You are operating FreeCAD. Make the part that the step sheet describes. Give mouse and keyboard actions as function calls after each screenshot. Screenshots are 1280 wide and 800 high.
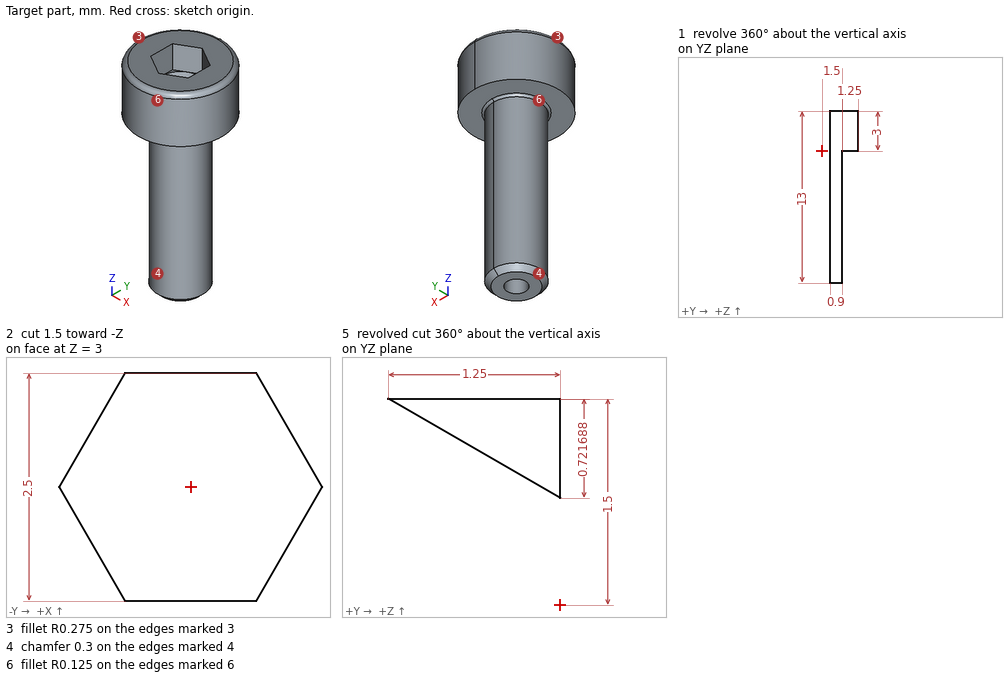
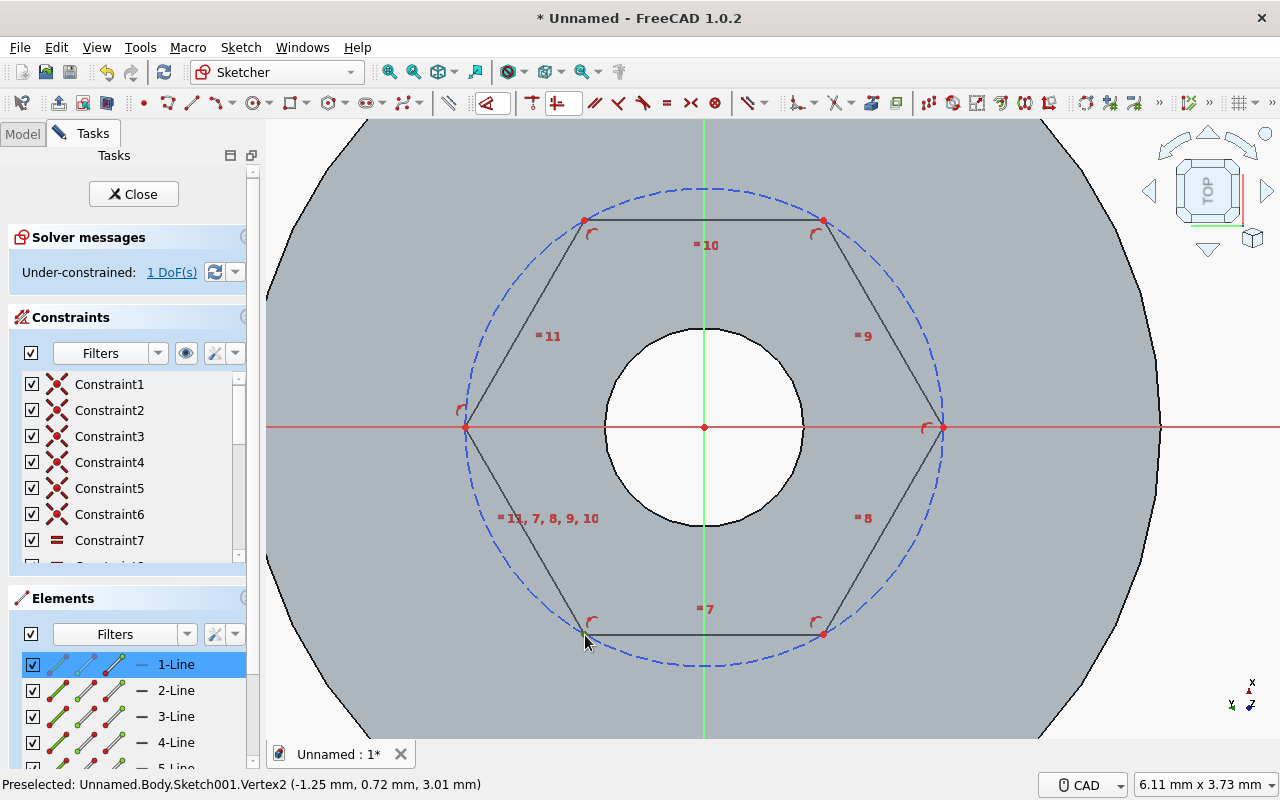
click(824, 220)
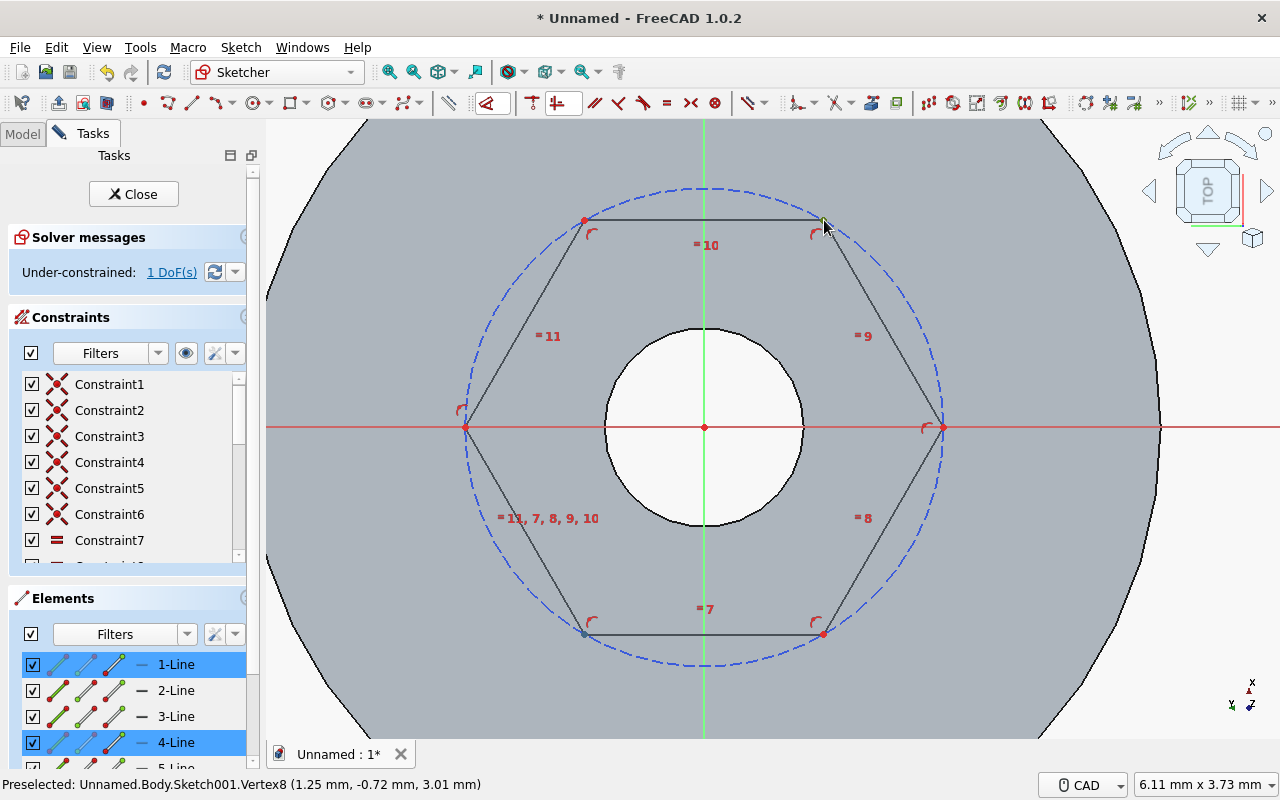
click(504, 104)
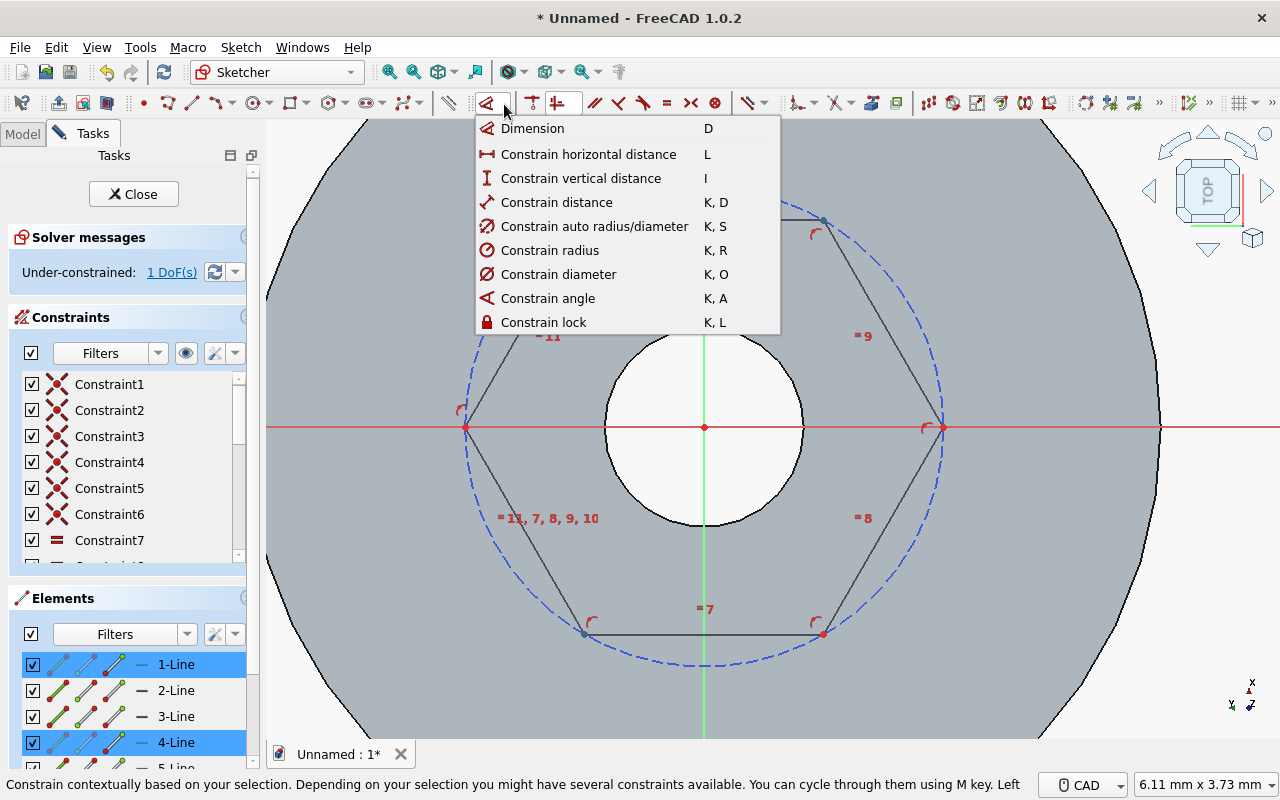
click(628, 178)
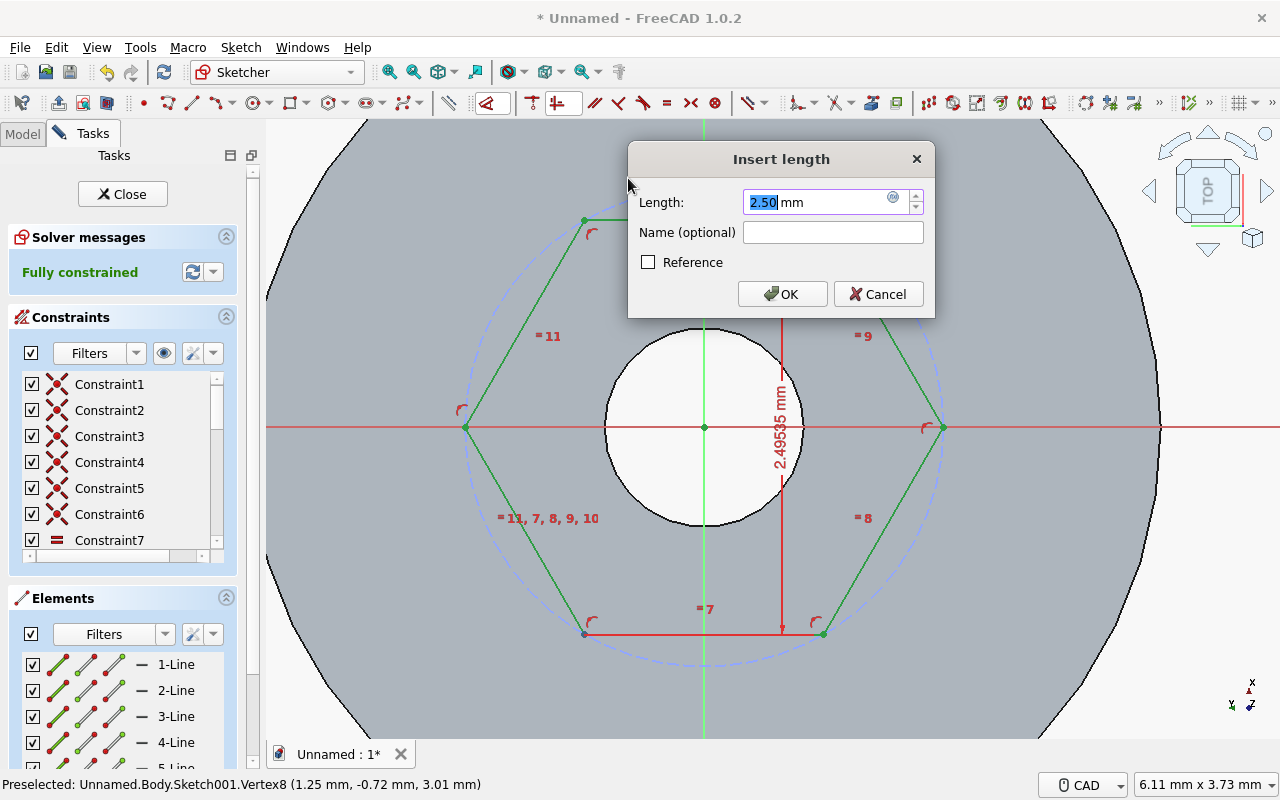
text(2.5)
key(Return)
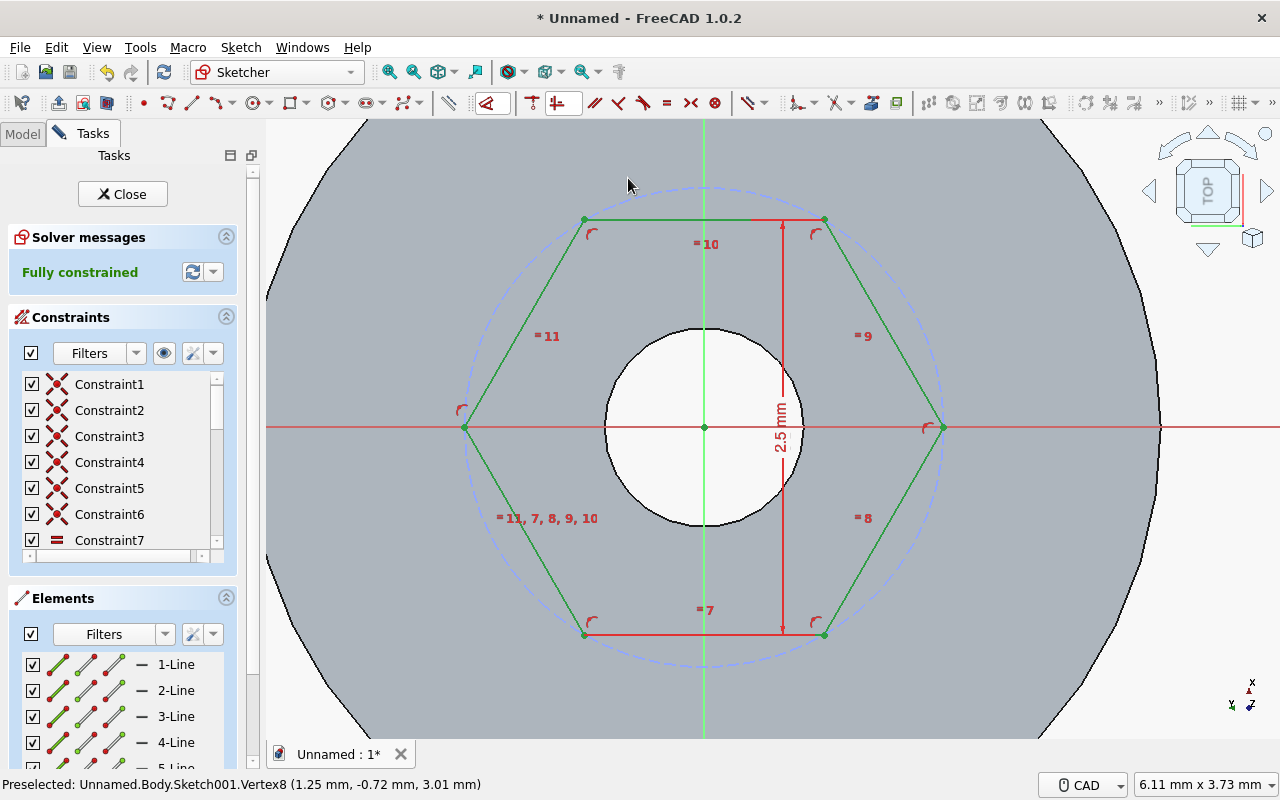
click(123, 194)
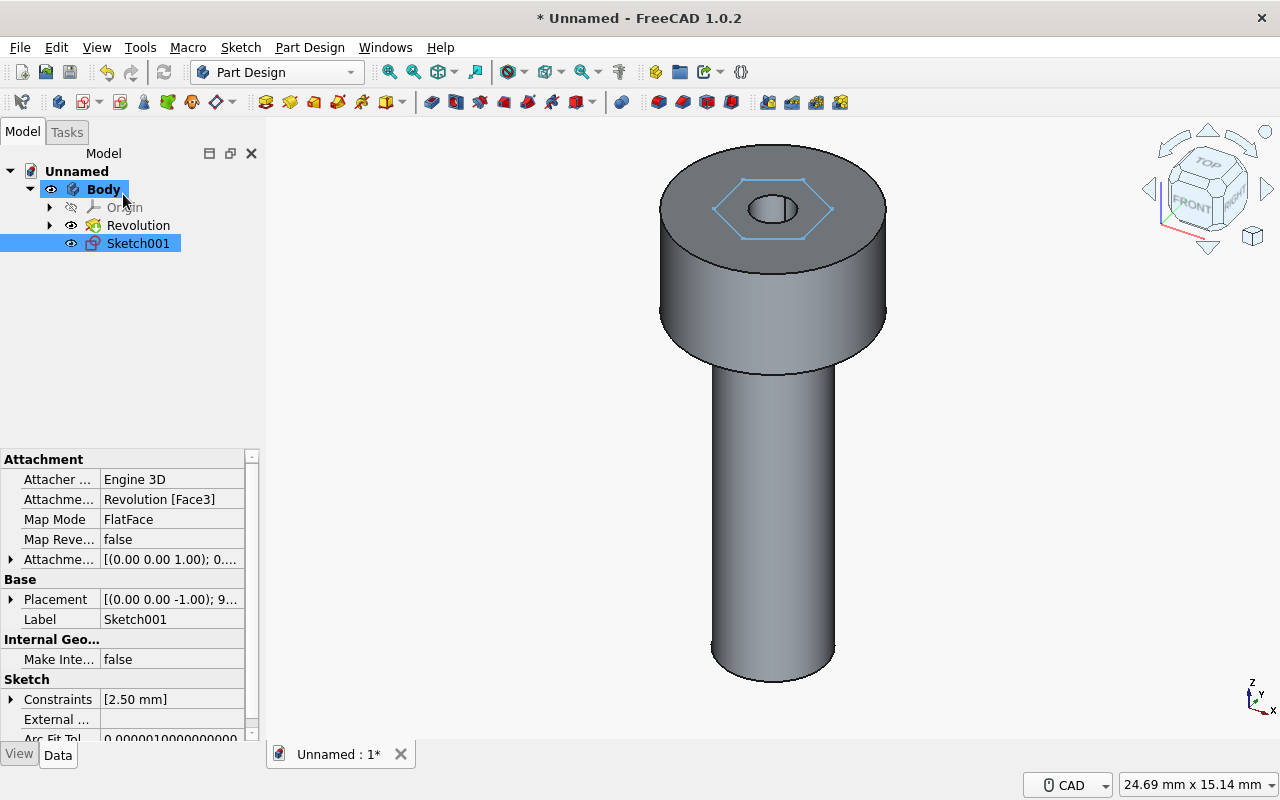
click(432, 102)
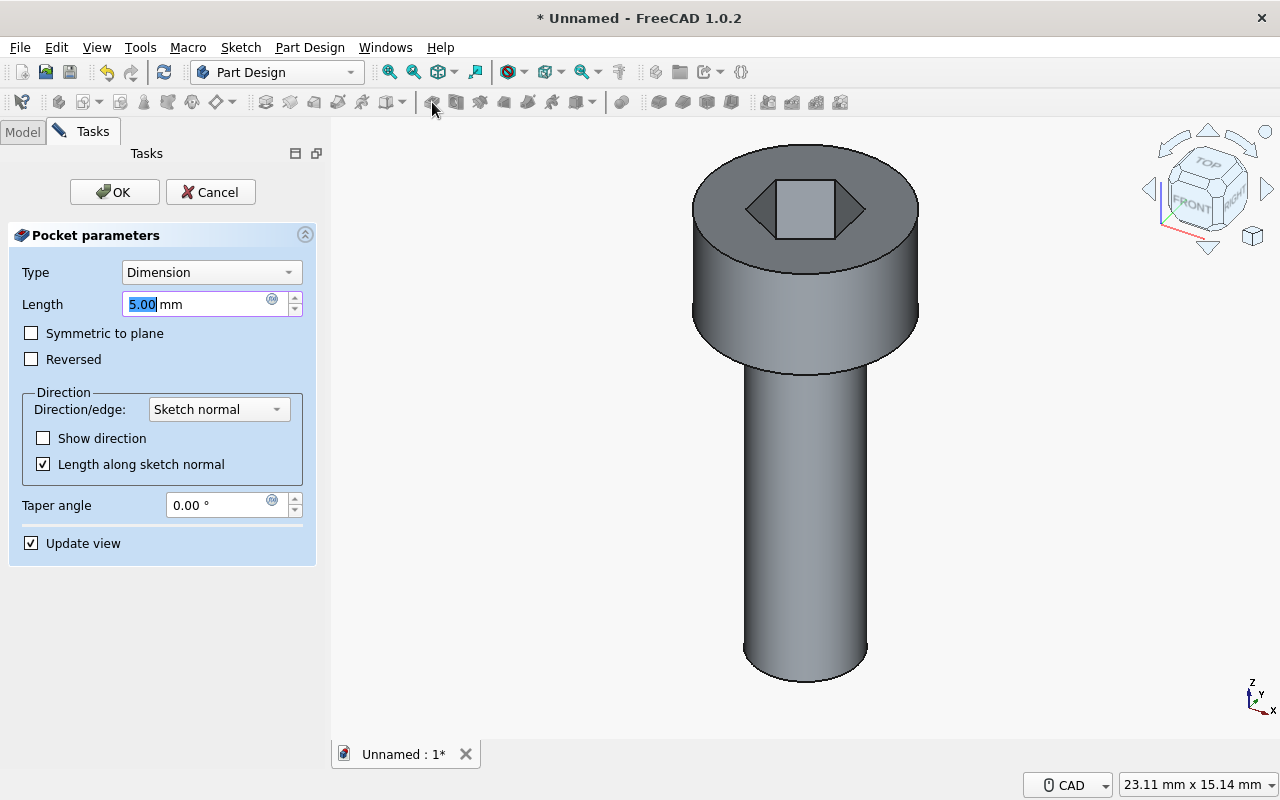
text(1.5)
key(Tab)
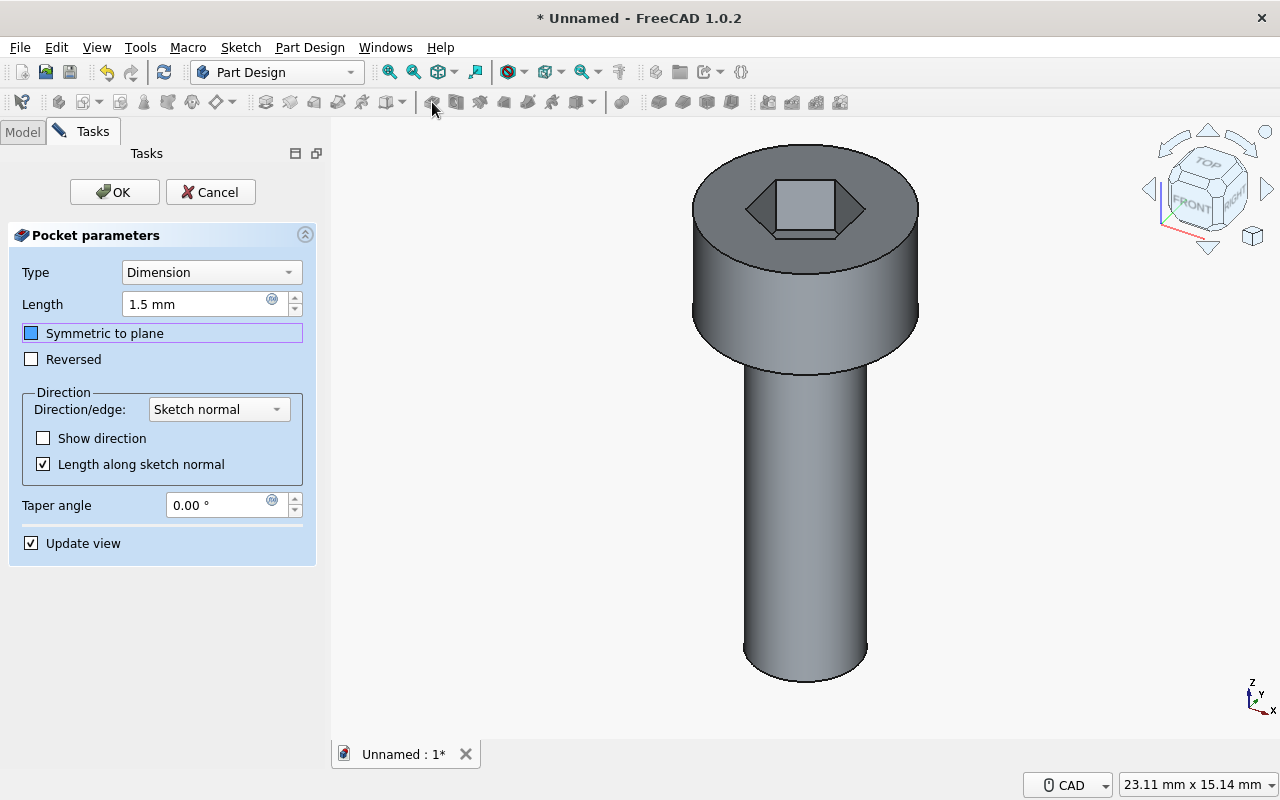
click(115, 192)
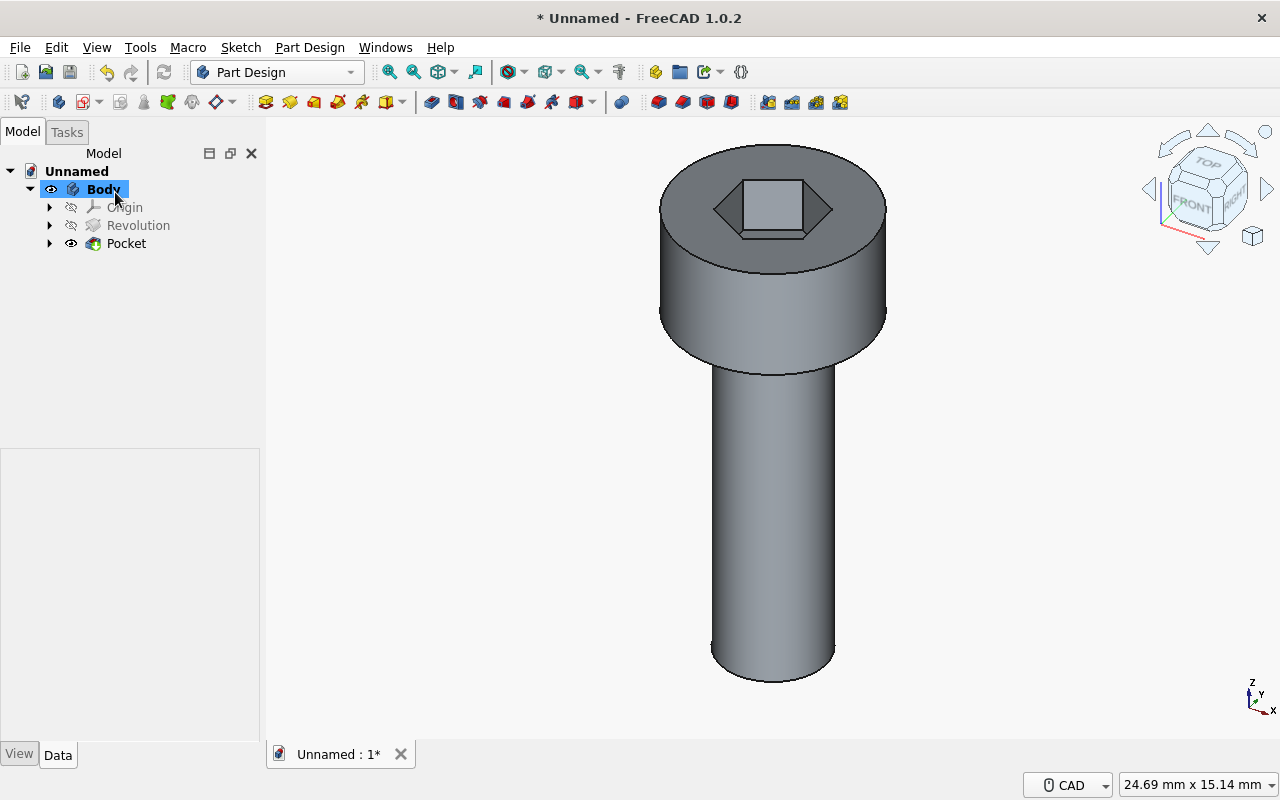
click(717, 264)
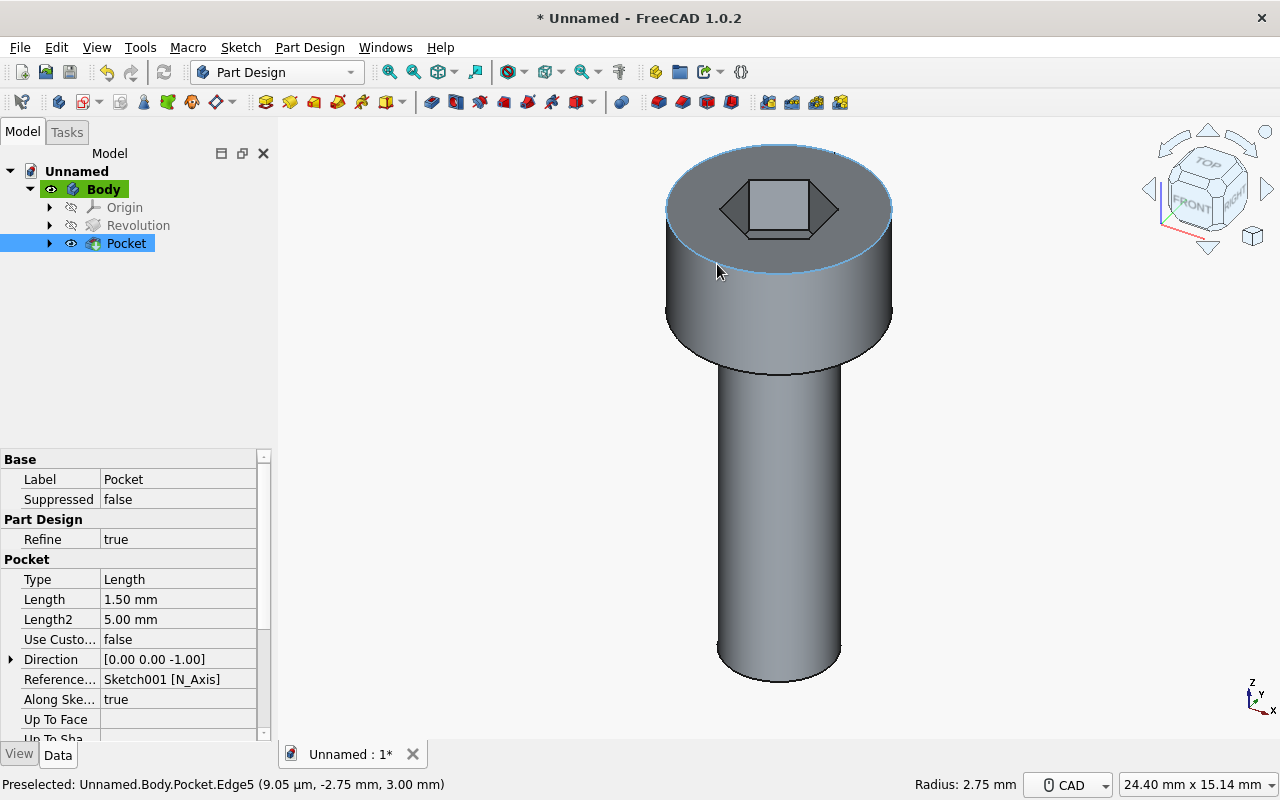
click(660, 102)